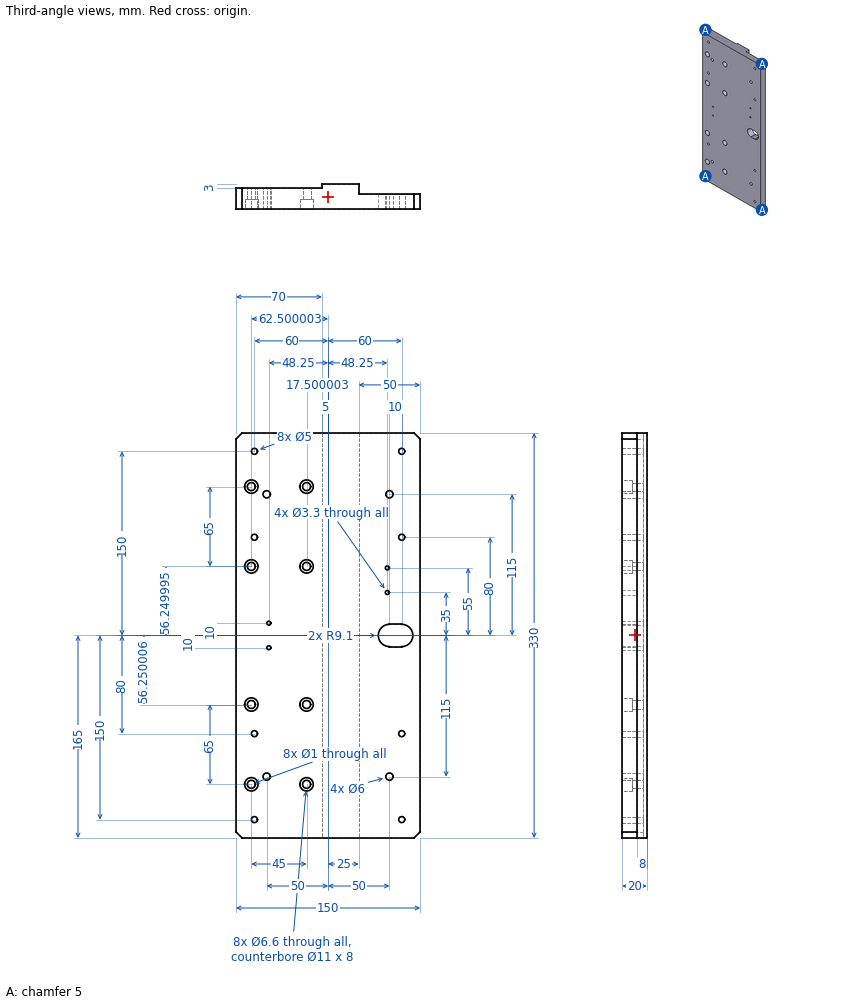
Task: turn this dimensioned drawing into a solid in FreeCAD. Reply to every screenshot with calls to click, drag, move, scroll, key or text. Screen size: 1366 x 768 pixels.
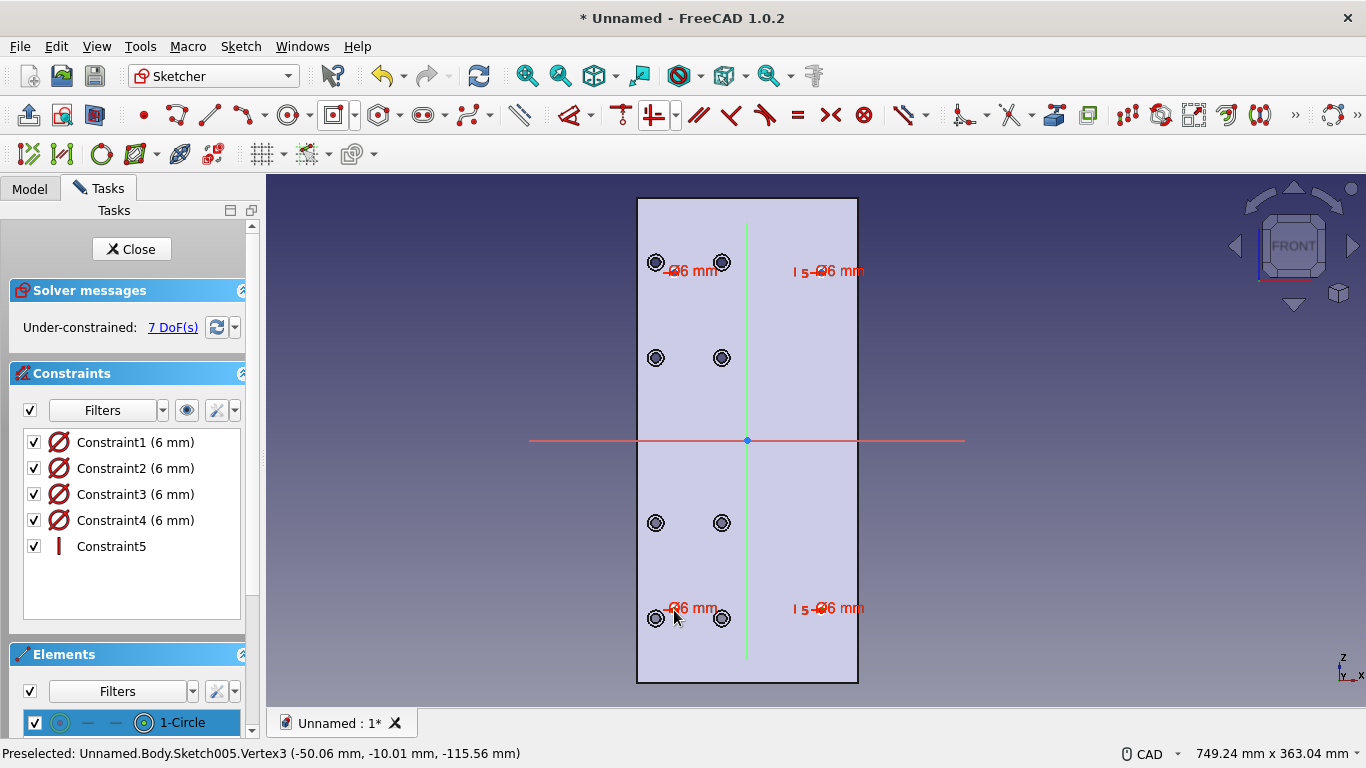
key(h)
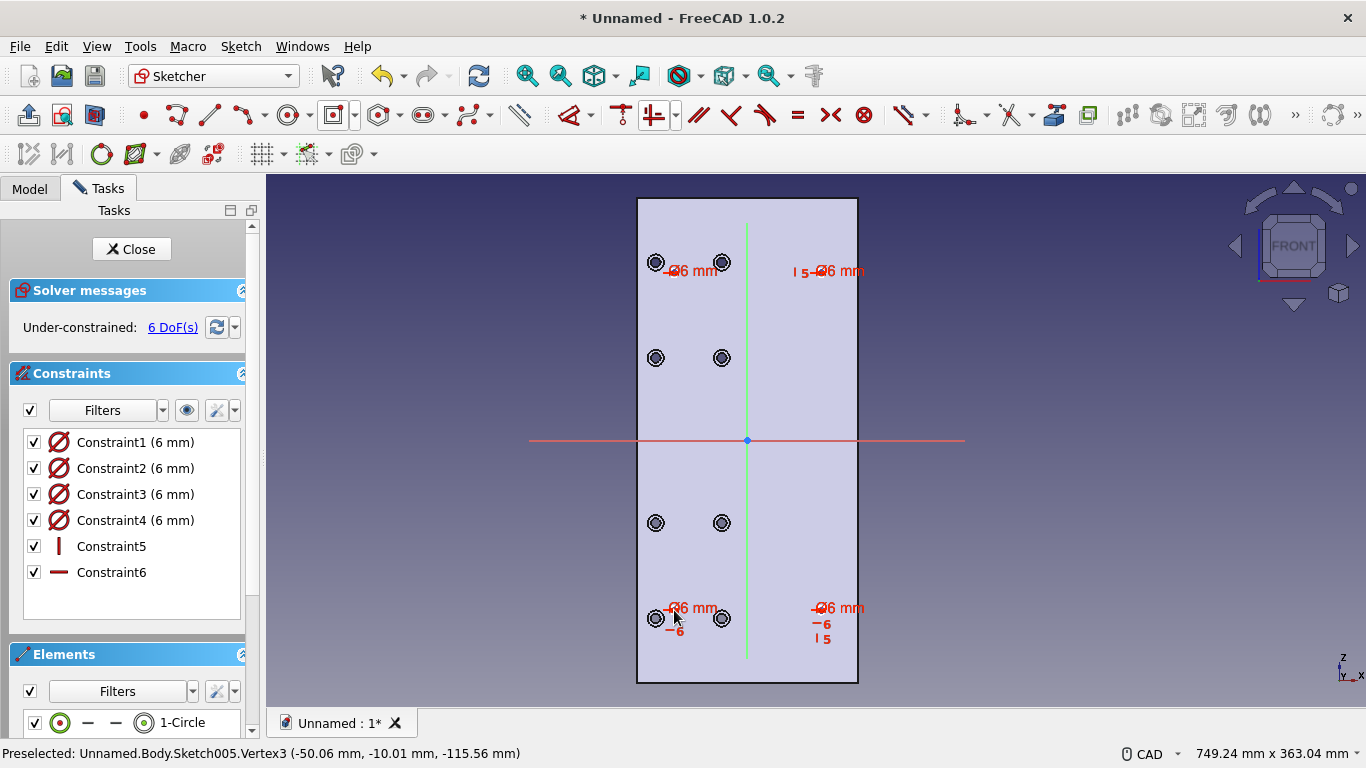
click(674, 610)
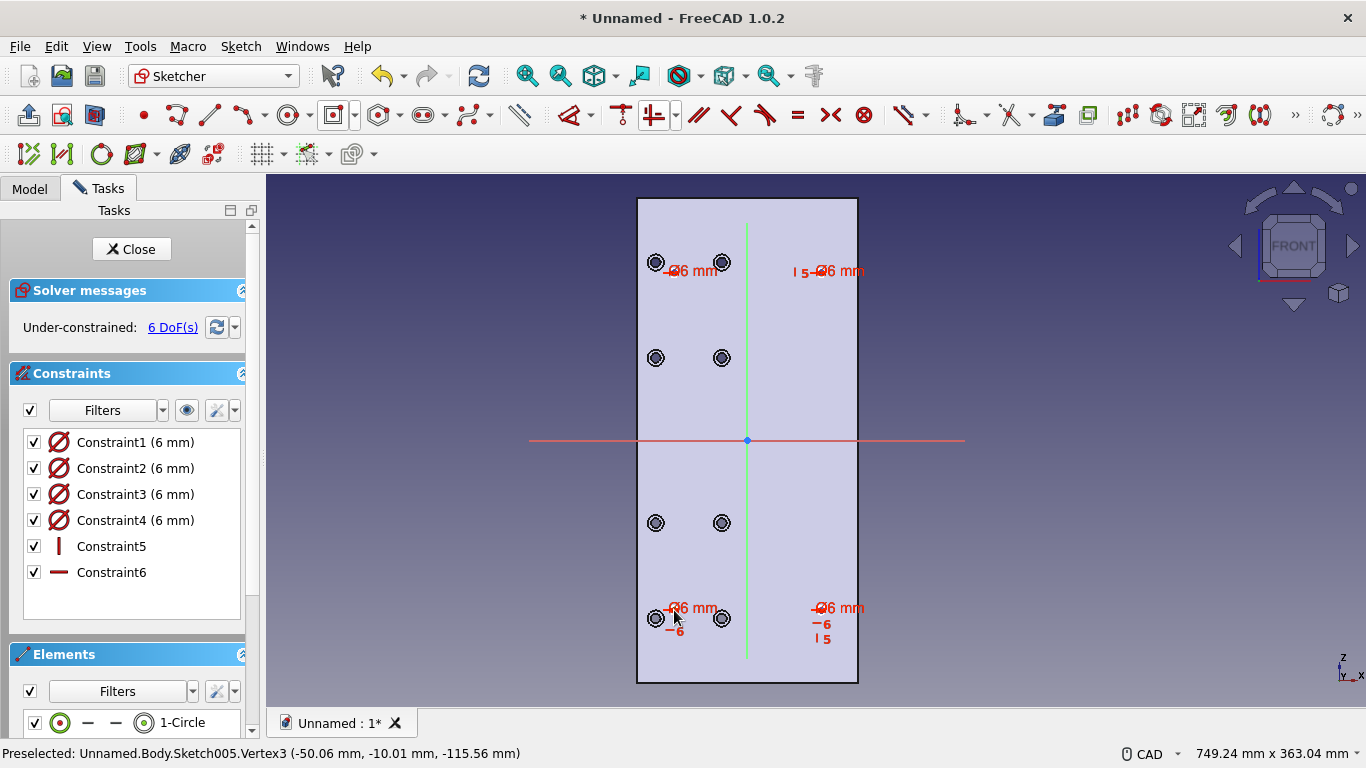
click(674, 273)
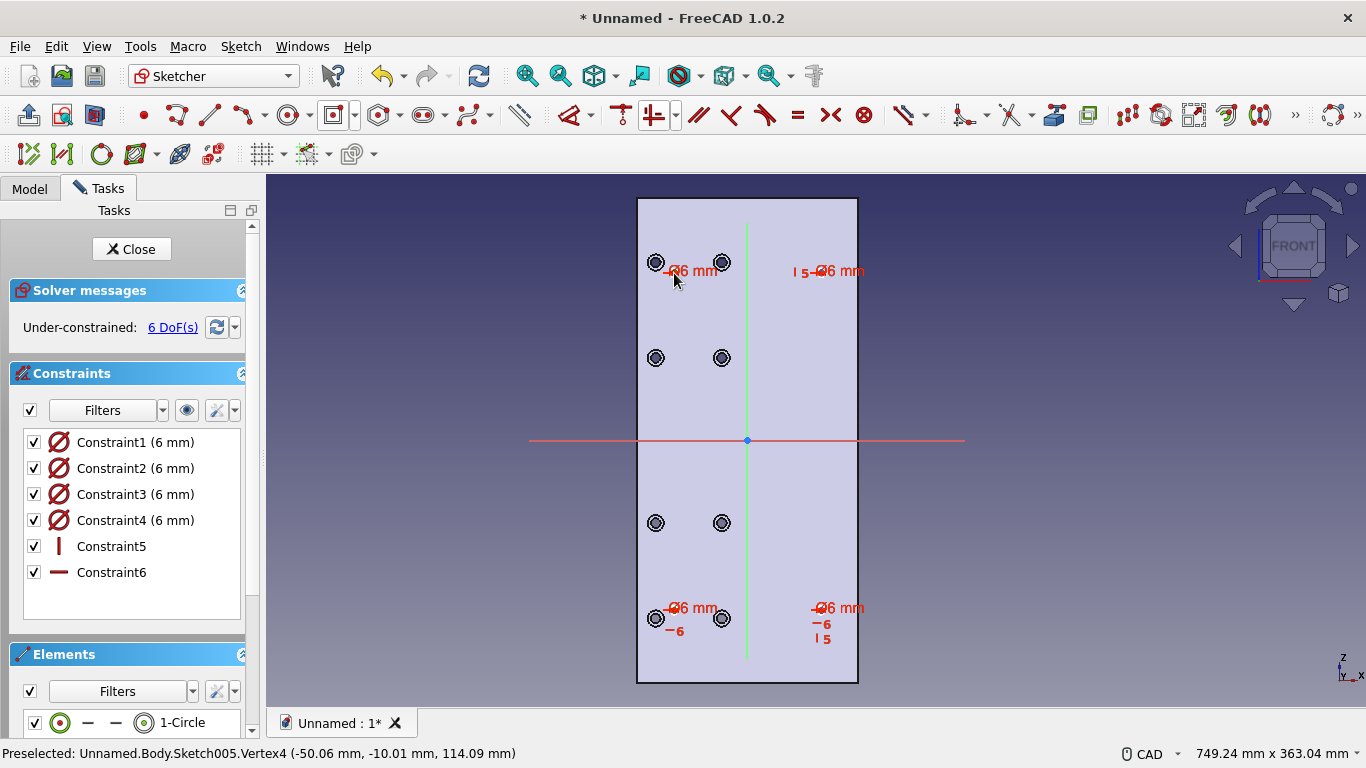
key(v)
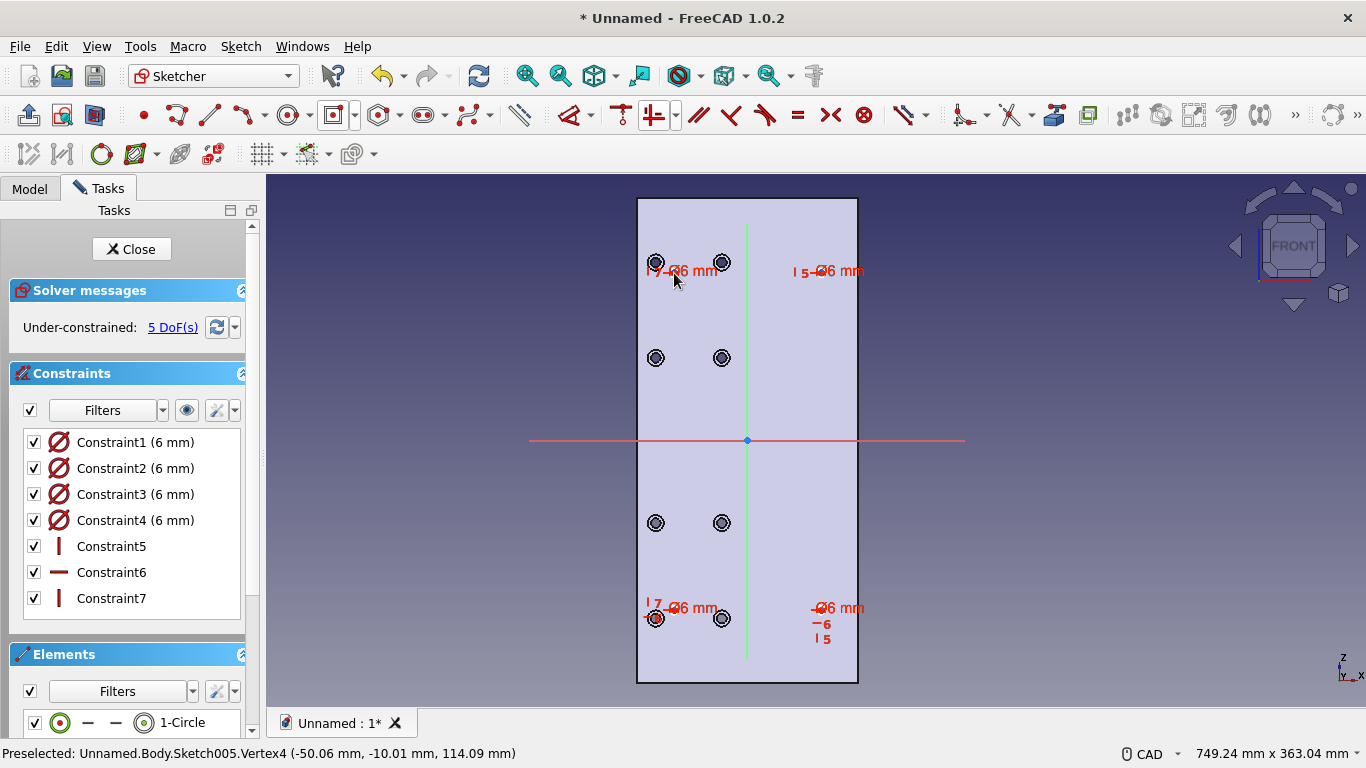
click(821, 273)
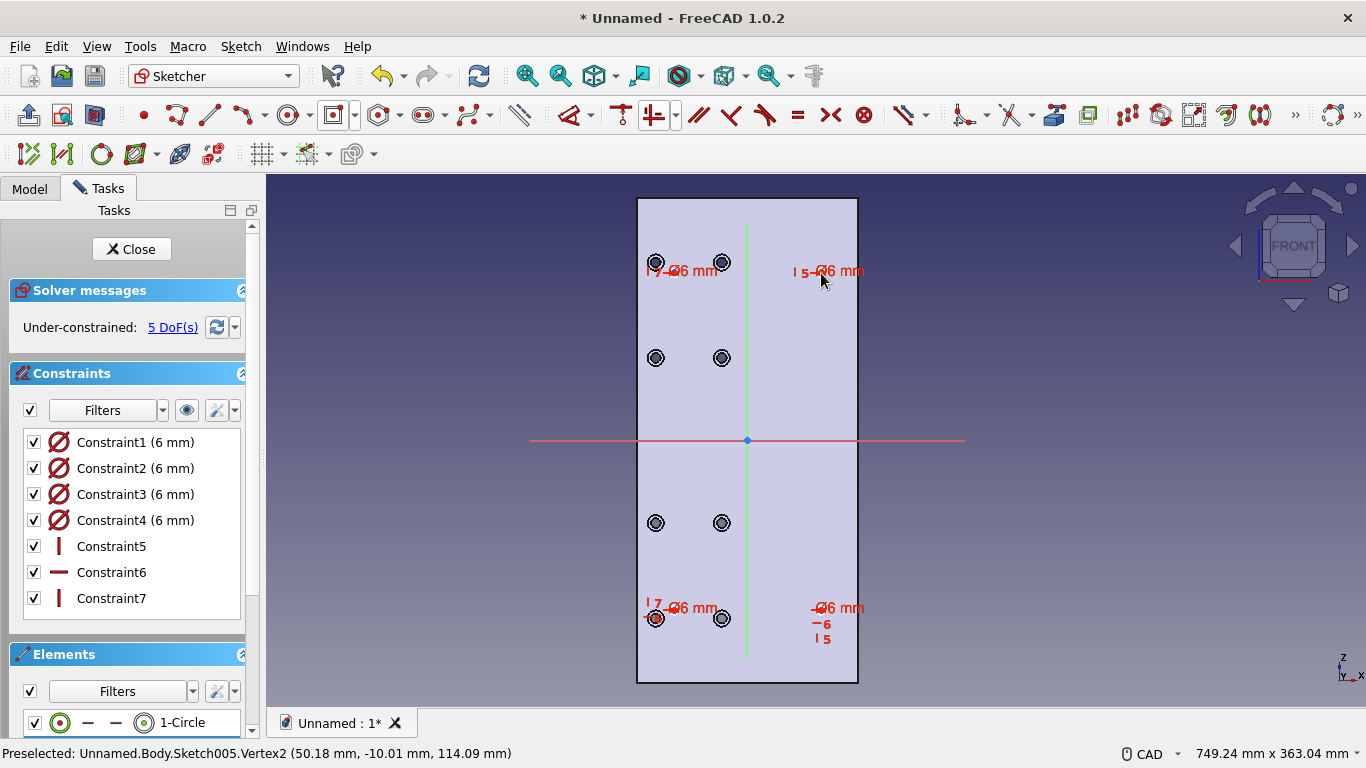
click(674, 273)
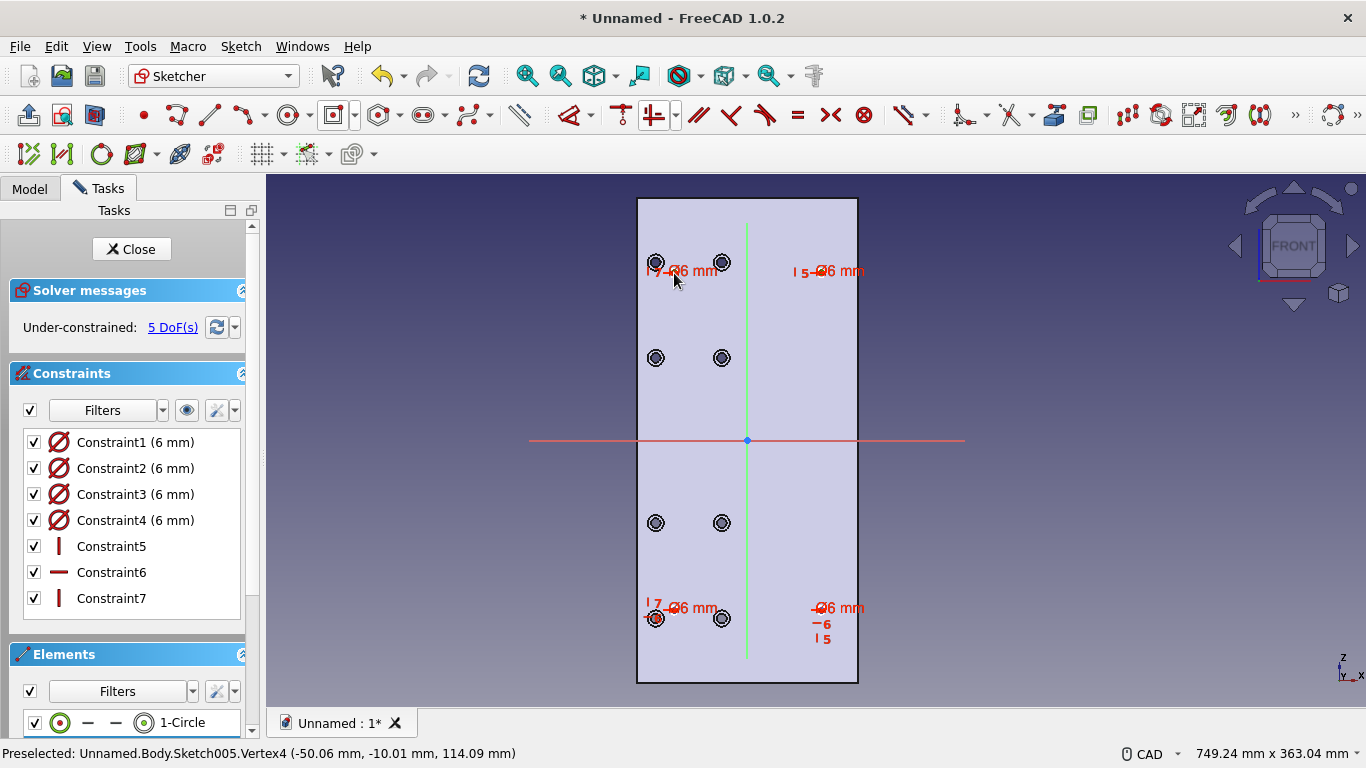
key(h)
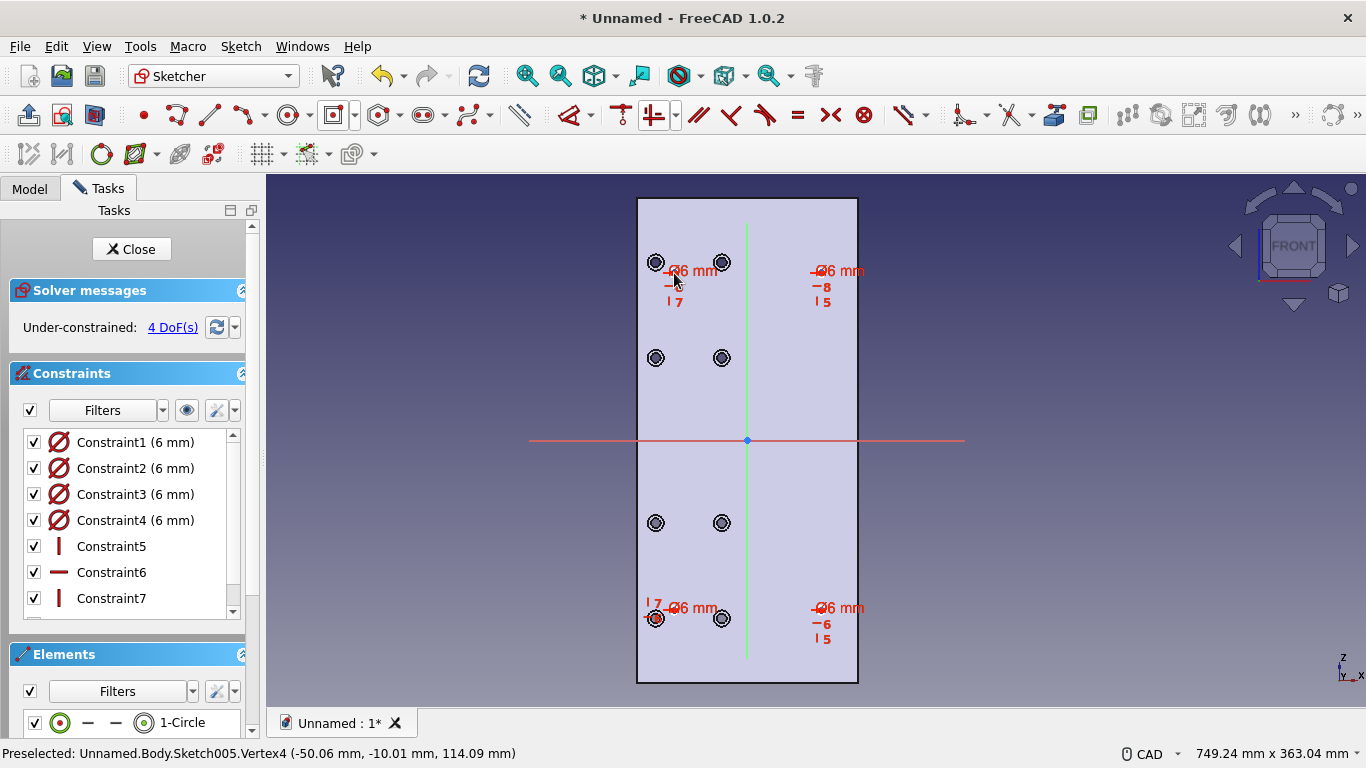
click(568, 116)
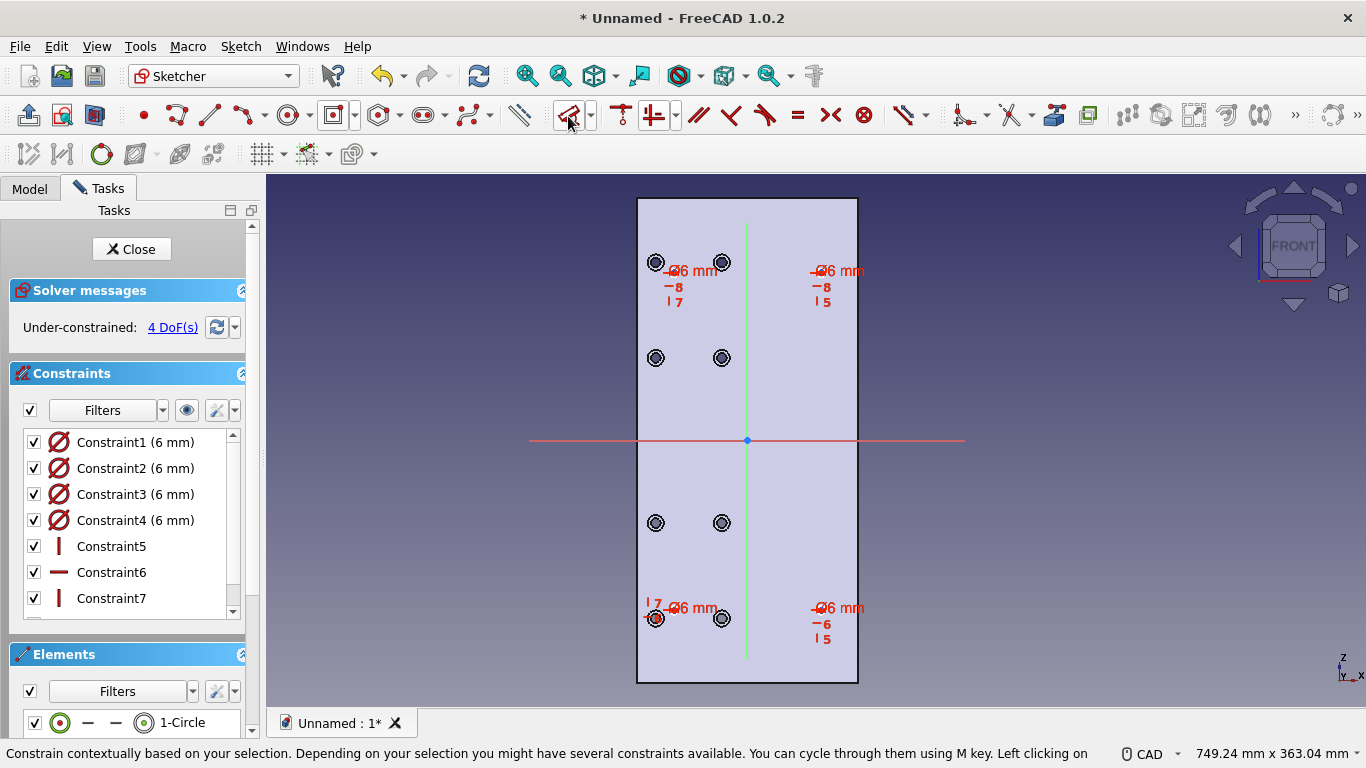
click(821, 610)
click(784, 644)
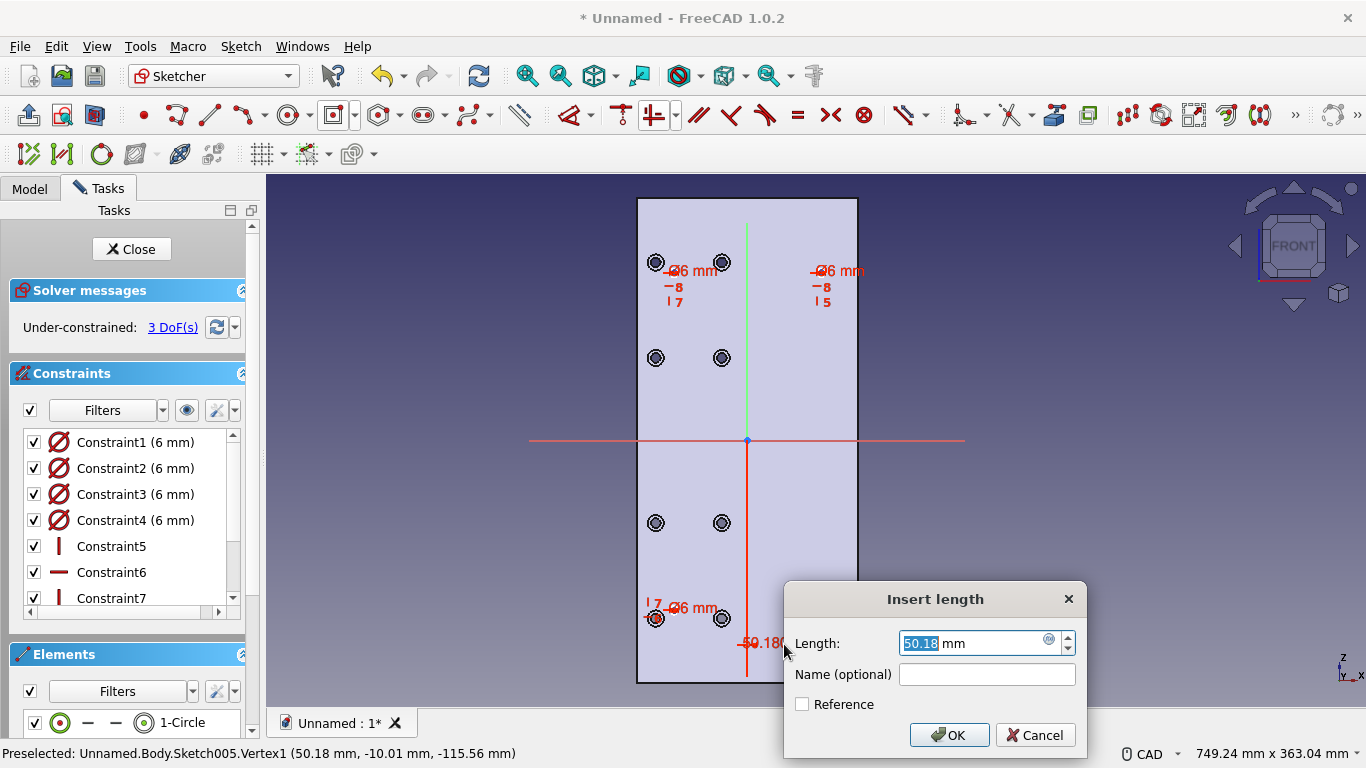
text(50)
key(Return)